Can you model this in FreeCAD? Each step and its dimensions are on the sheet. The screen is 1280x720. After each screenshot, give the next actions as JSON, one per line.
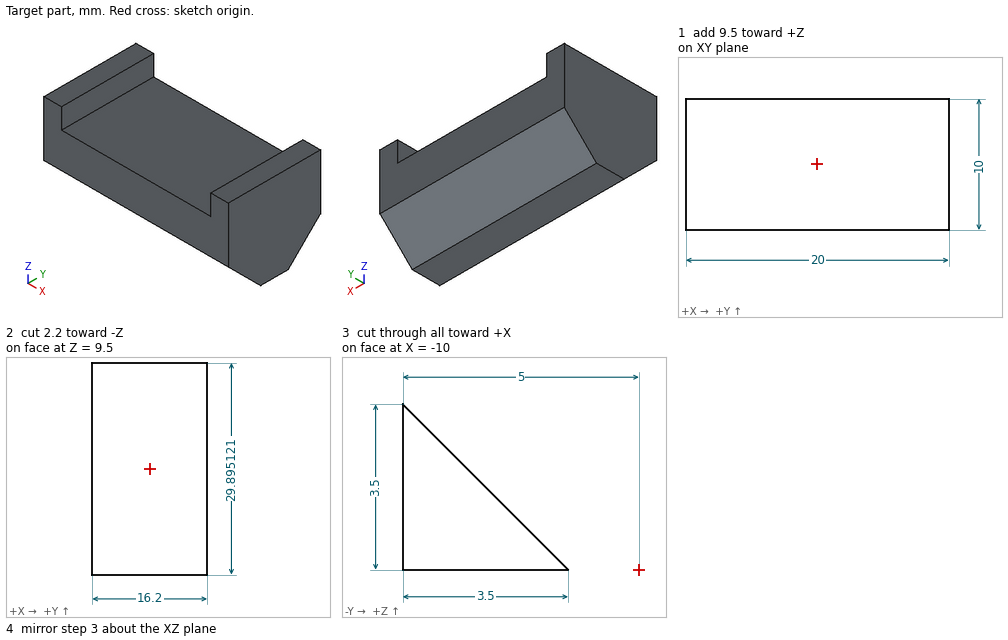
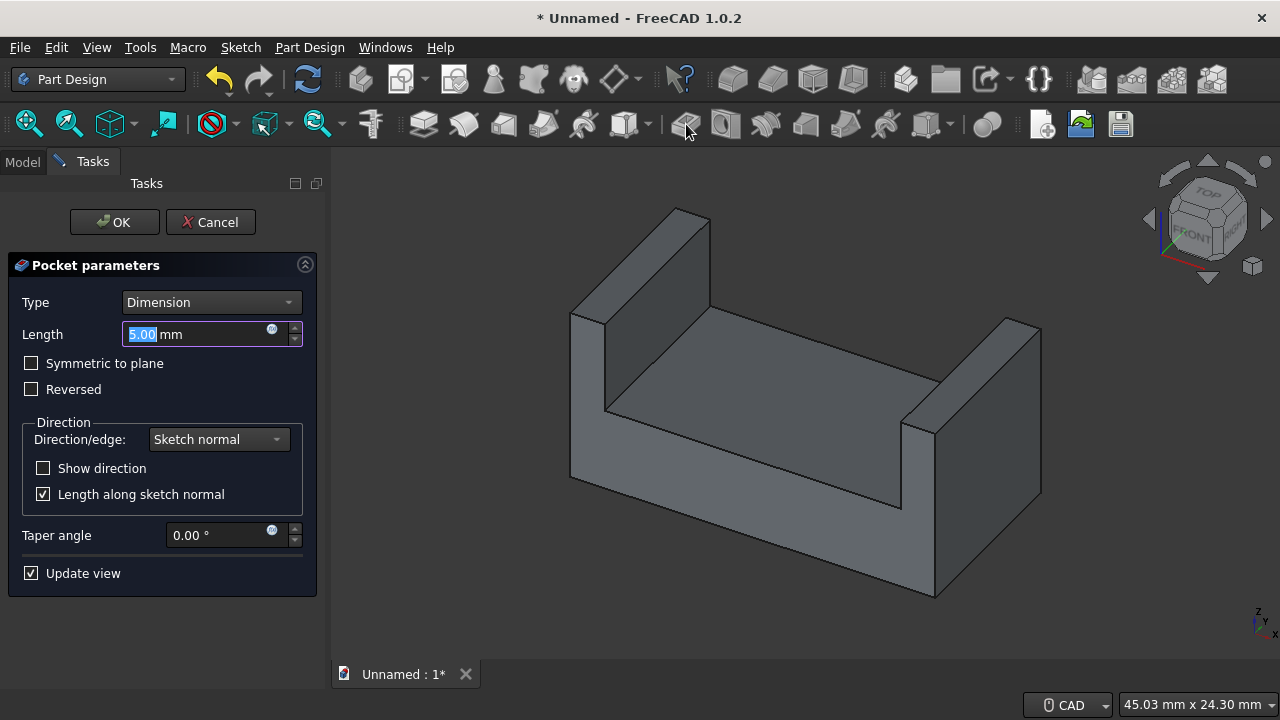
{"action": "type", "text": "2.2"}
{"action": "key", "text": "Tab"}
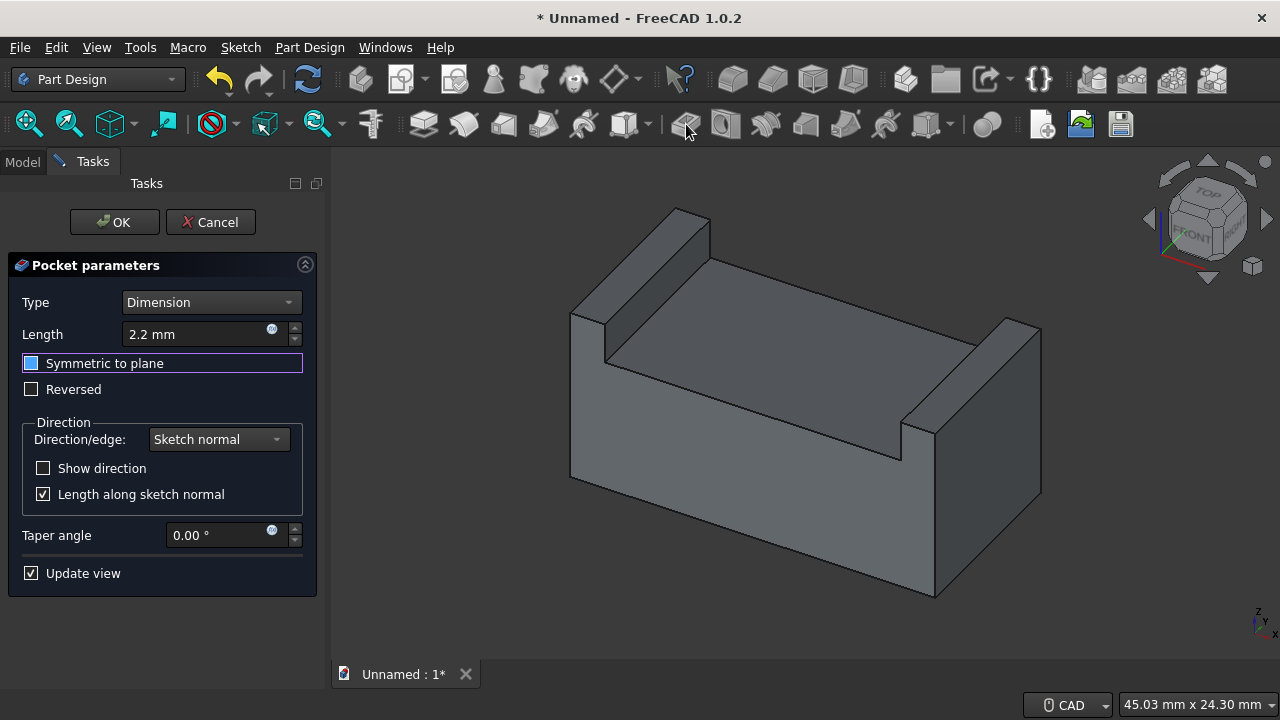
{"action": "left_click", "coordinate": [115, 222]}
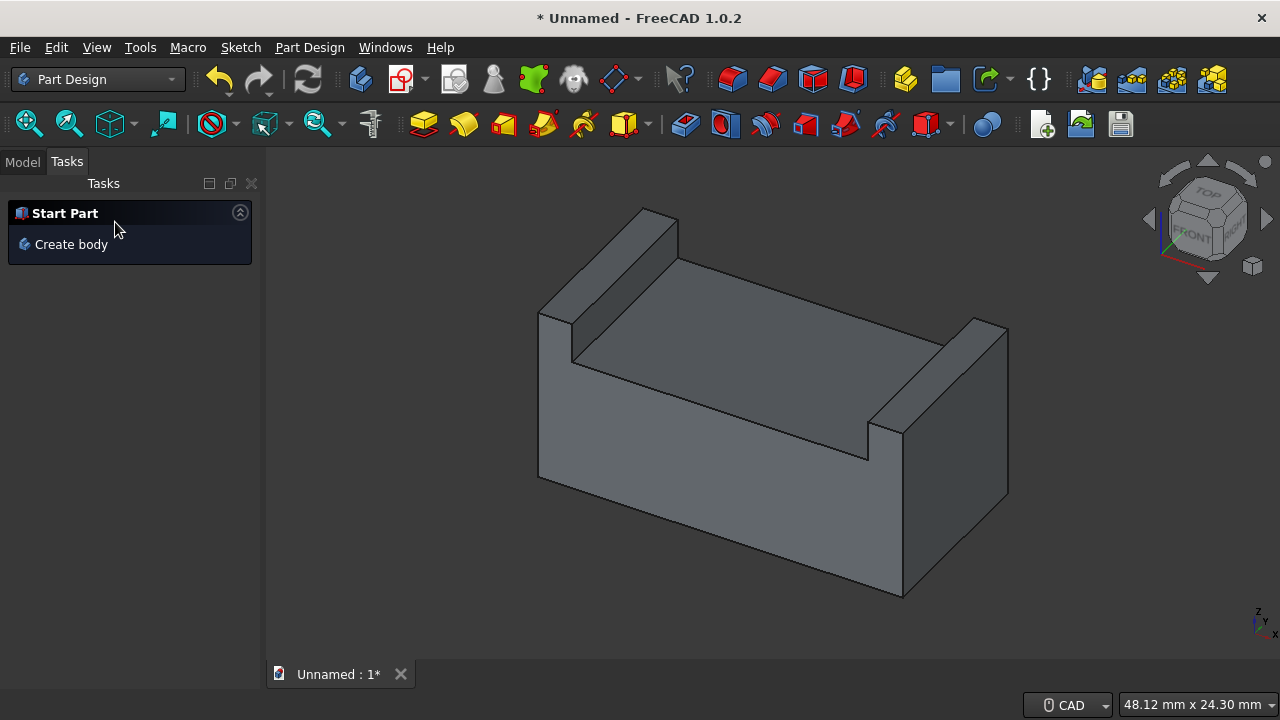
{"action": "key", "text": "6"}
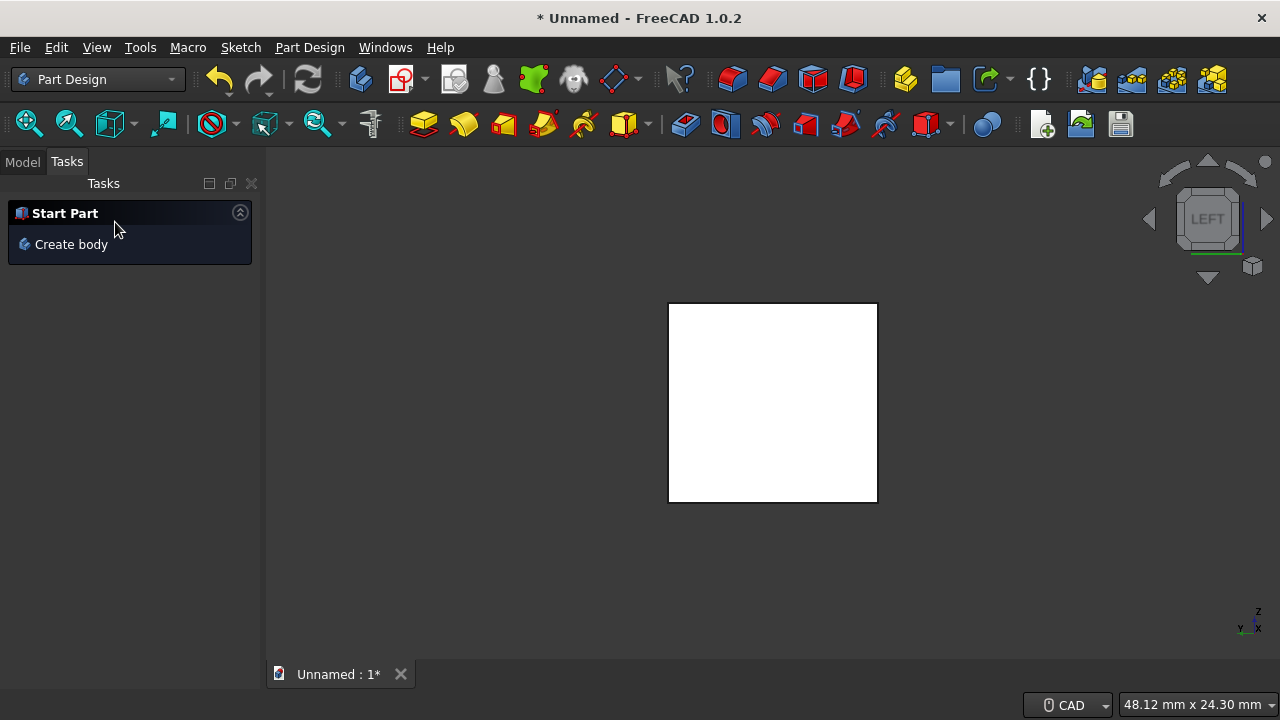
{"action": "key", "text": "v f"}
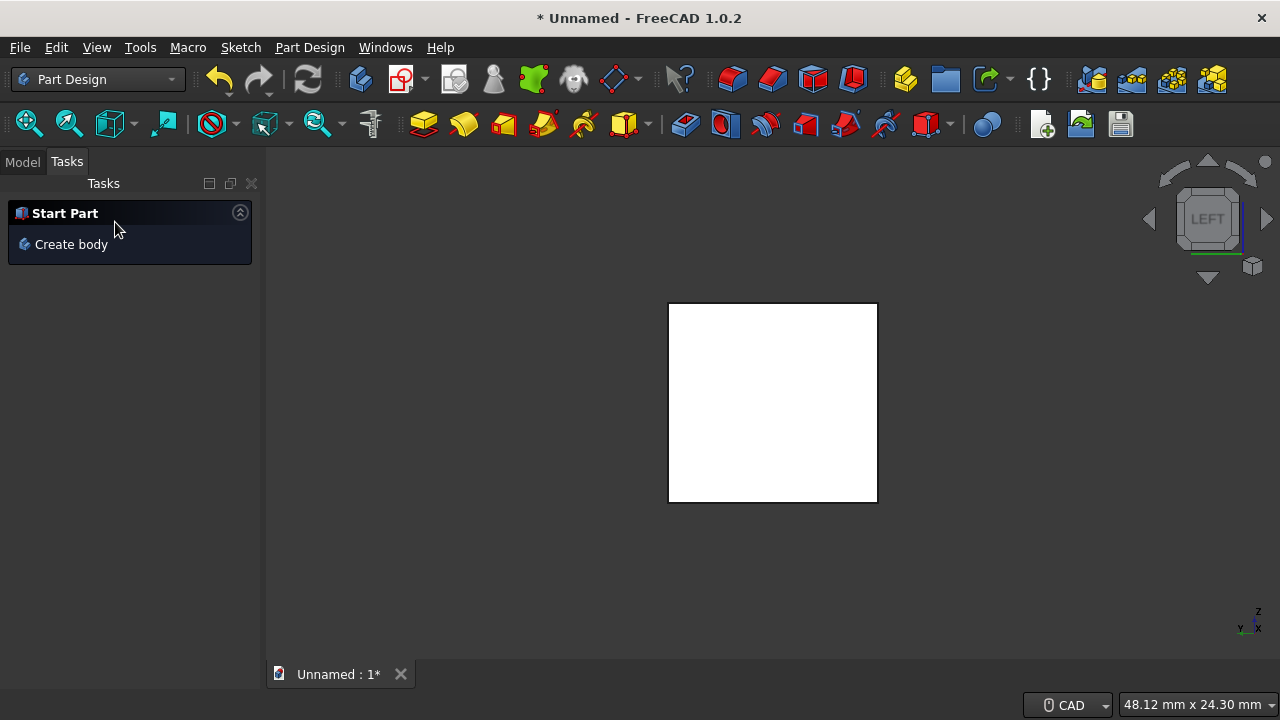
{"action": "left_click", "coordinate": [773, 402]}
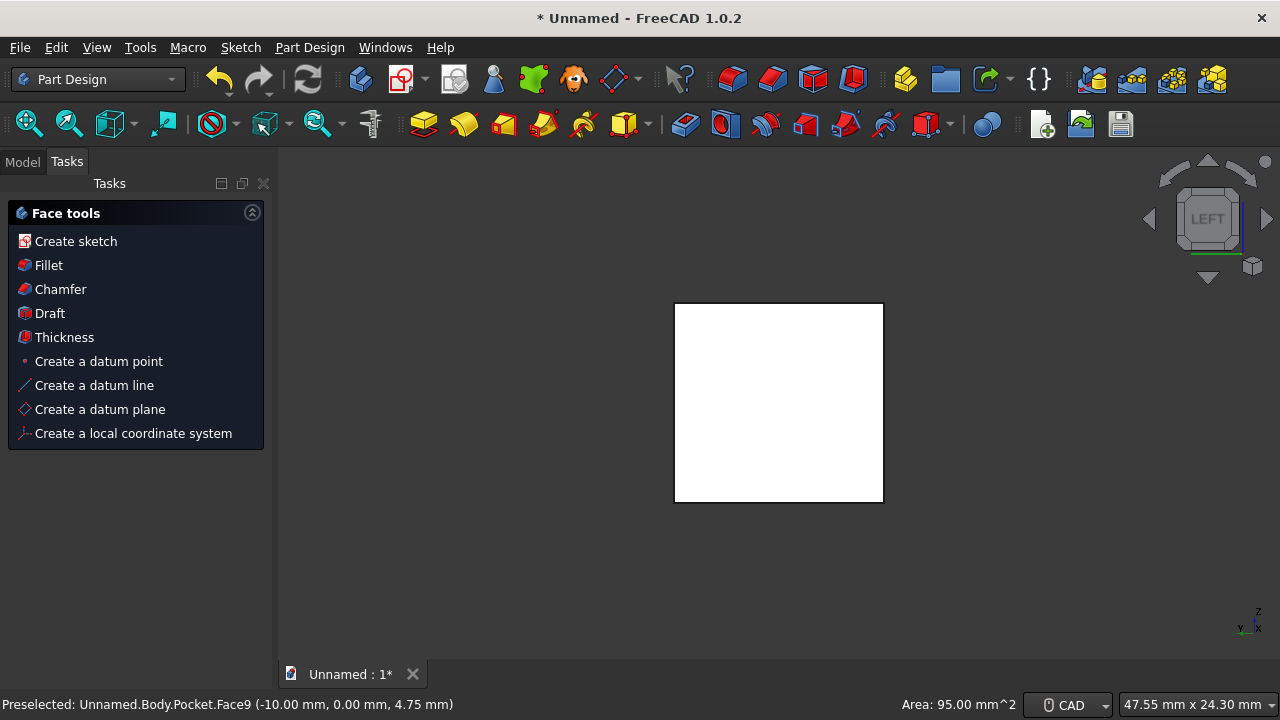
{"action": "left_click", "coordinate": [402, 80]}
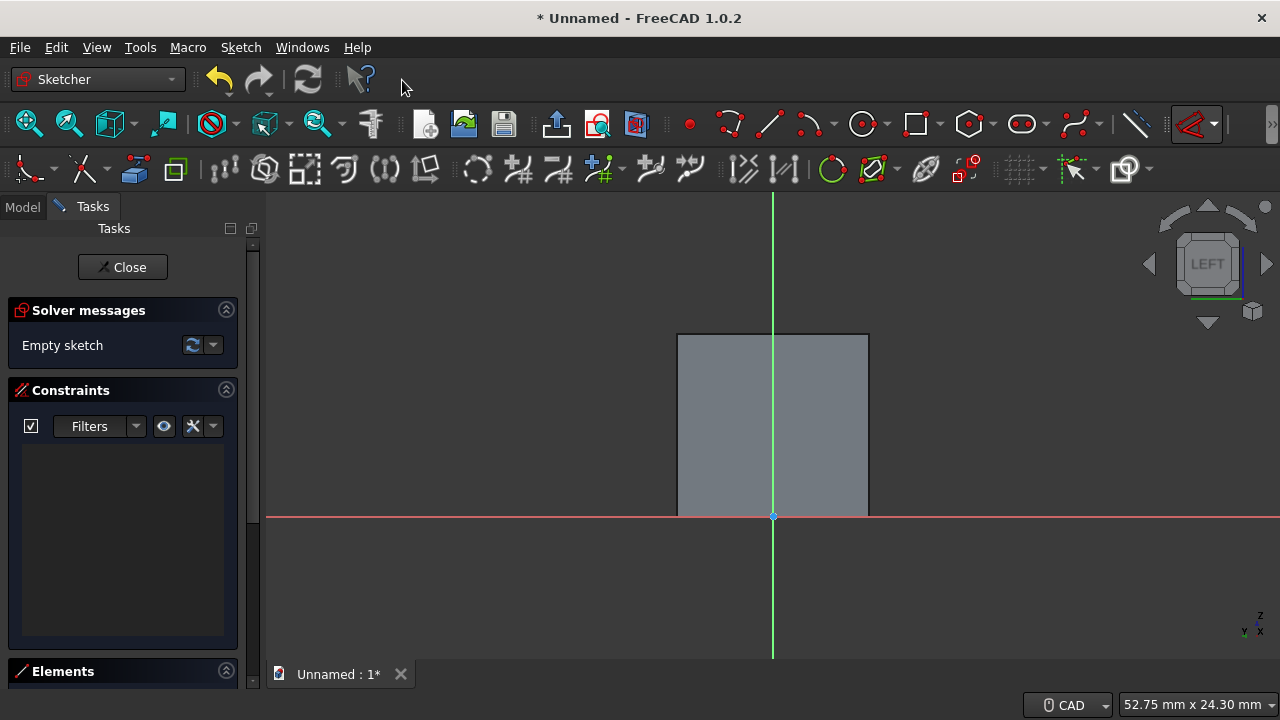
{"action": "scroll", "coordinate": [732, 502], "scroll_direction": "up", "scroll_amount": 7}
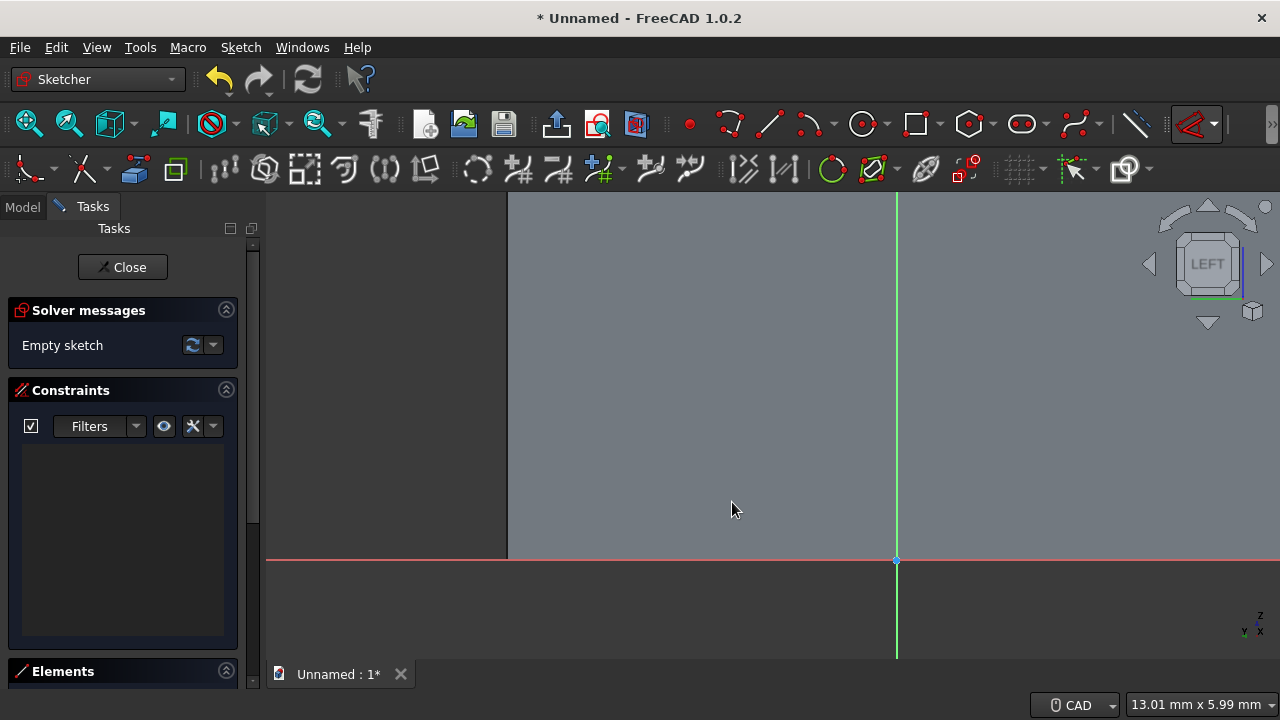
{"action": "left_click", "coordinate": [730, 124]}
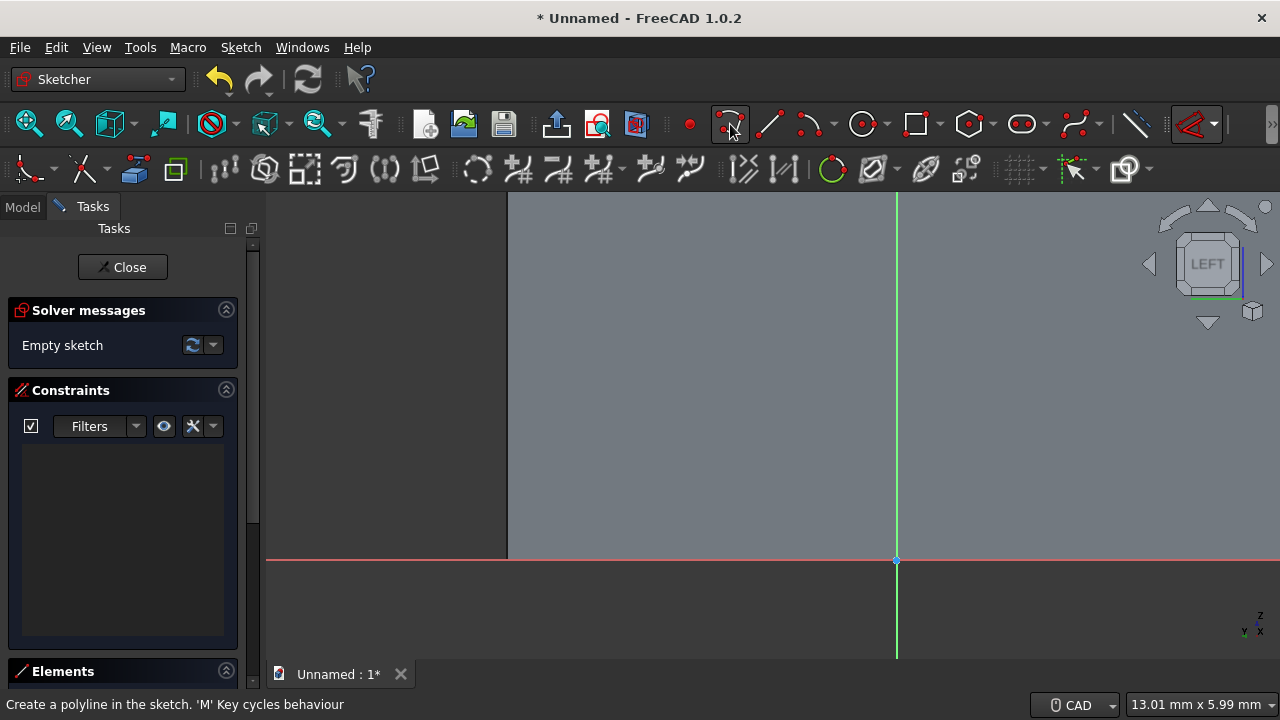
{"action": "left_click", "coordinate": [780, 560]}
{"action": "left_click", "coordinate": [507, 287]}
{"action": "left_click", "coordinate": [507, 551]}
{"action": "left_click", "coordinate": [780, 560]}
{"action": "key", "text": "Escape"}
{"action": "key", "text": "Escape"}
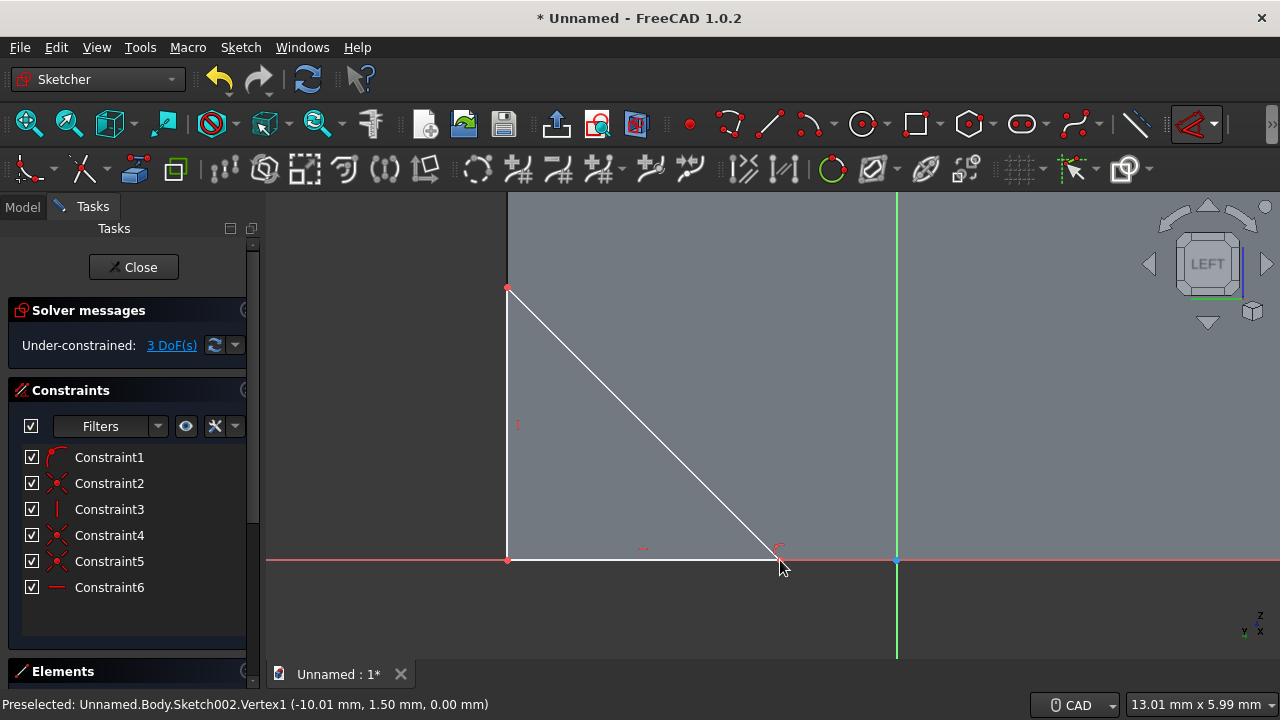
{"action": "left_click", "coordinate": [507, 288]}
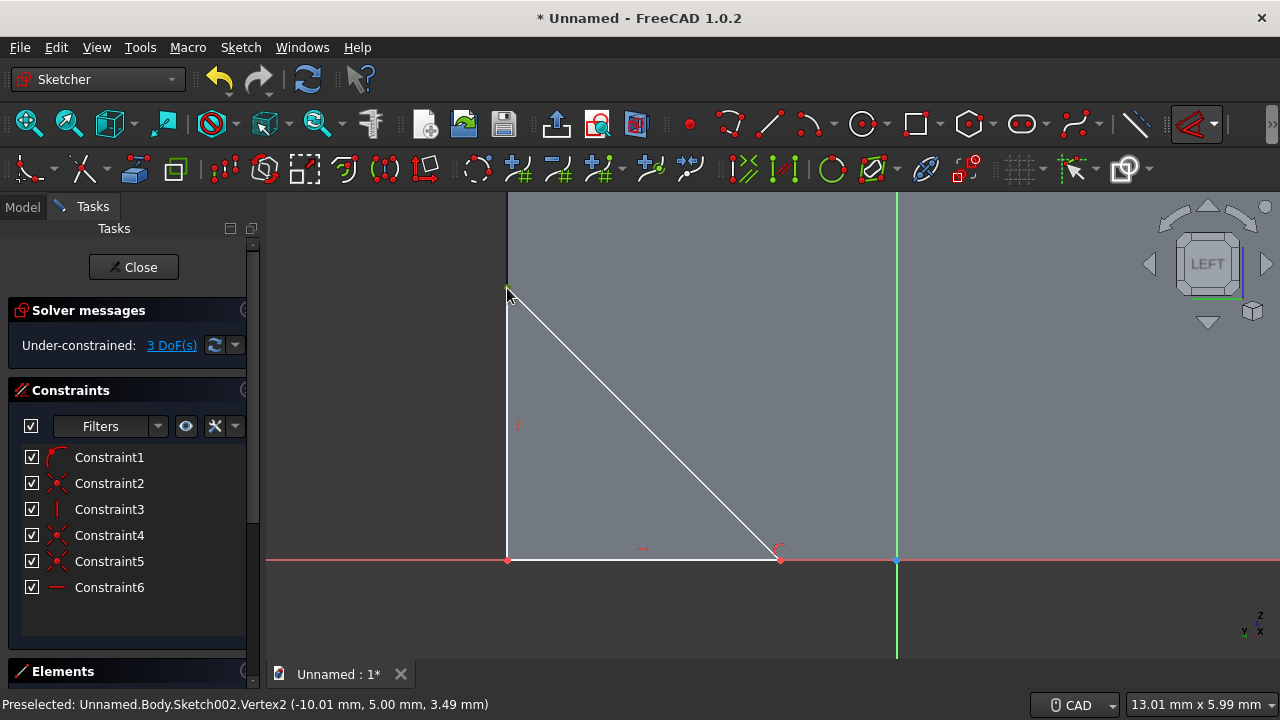
{"action": "key", "text": "l"}